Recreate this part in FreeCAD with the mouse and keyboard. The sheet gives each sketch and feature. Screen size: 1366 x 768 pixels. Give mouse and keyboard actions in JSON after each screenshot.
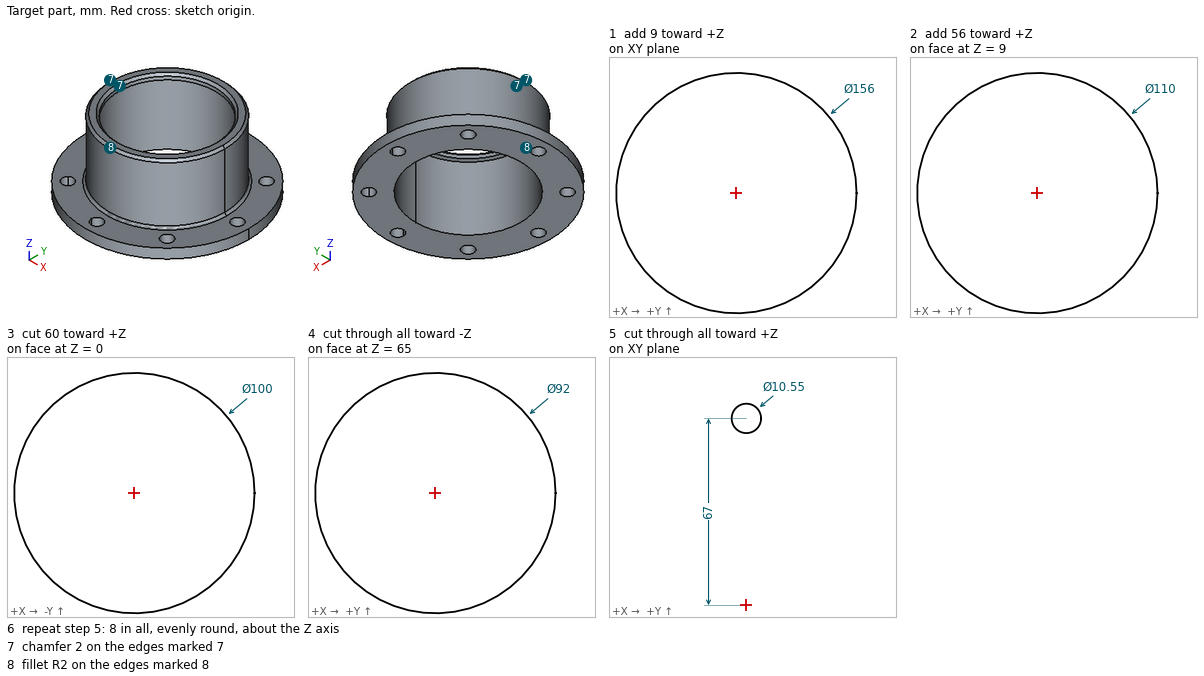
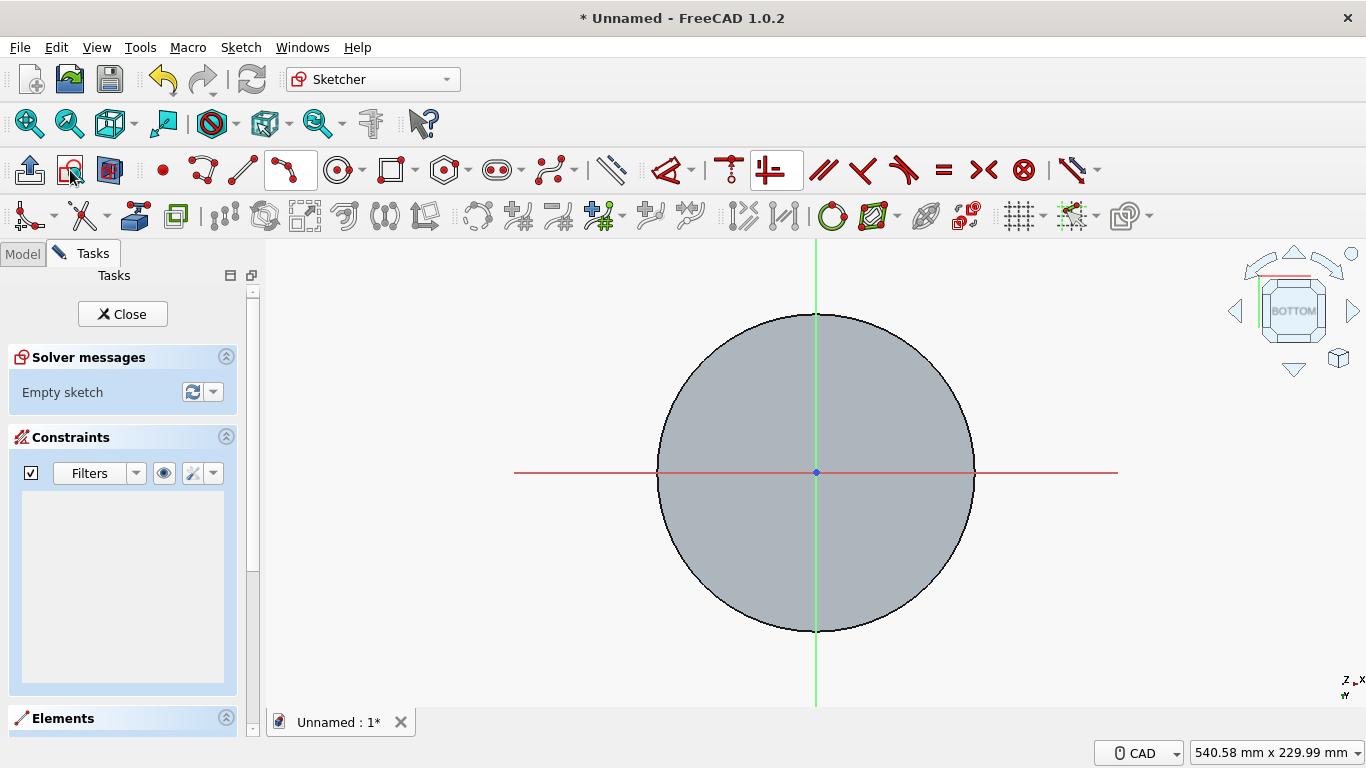
{"action": "scroll", "coordinate": [955, 473], "scroll_direction": "up", "scroll_amount": 2}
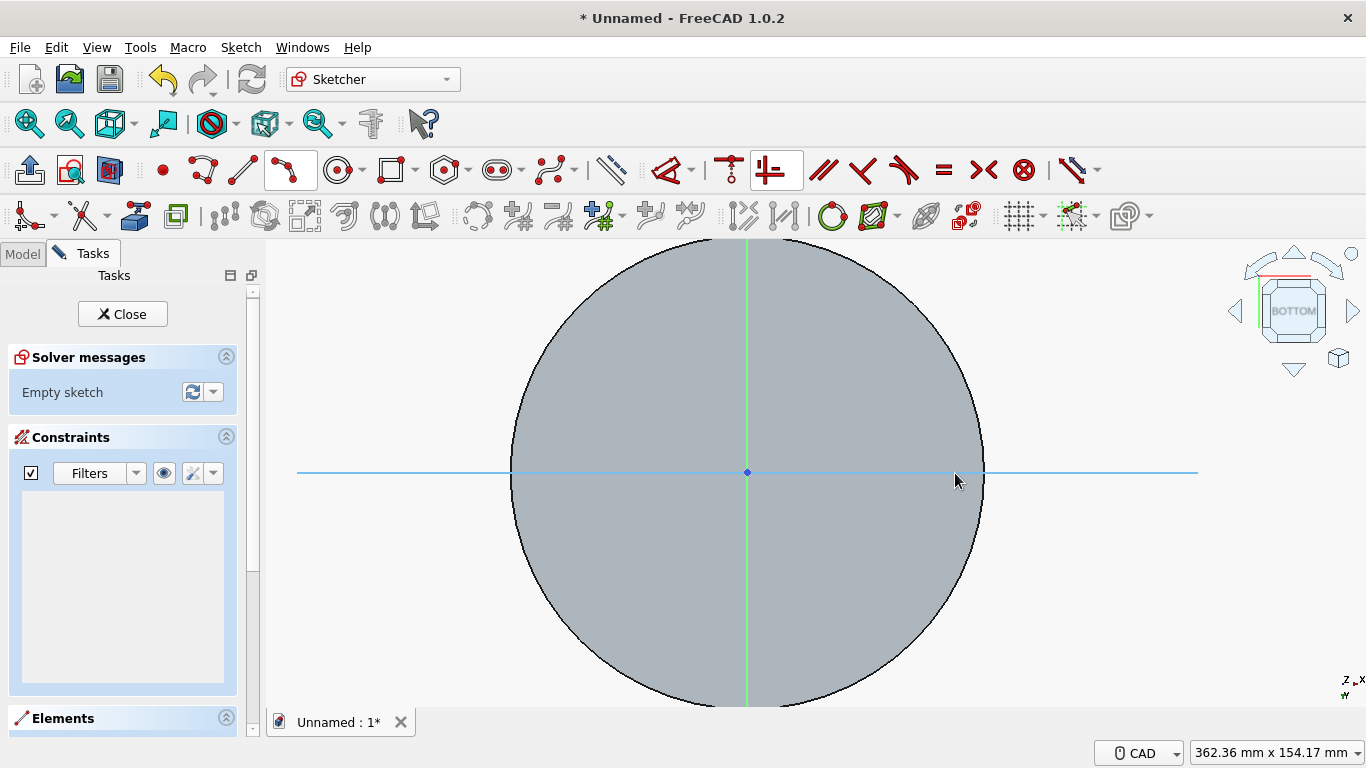
{"action": "left_click", "coordinate": [338, 170]}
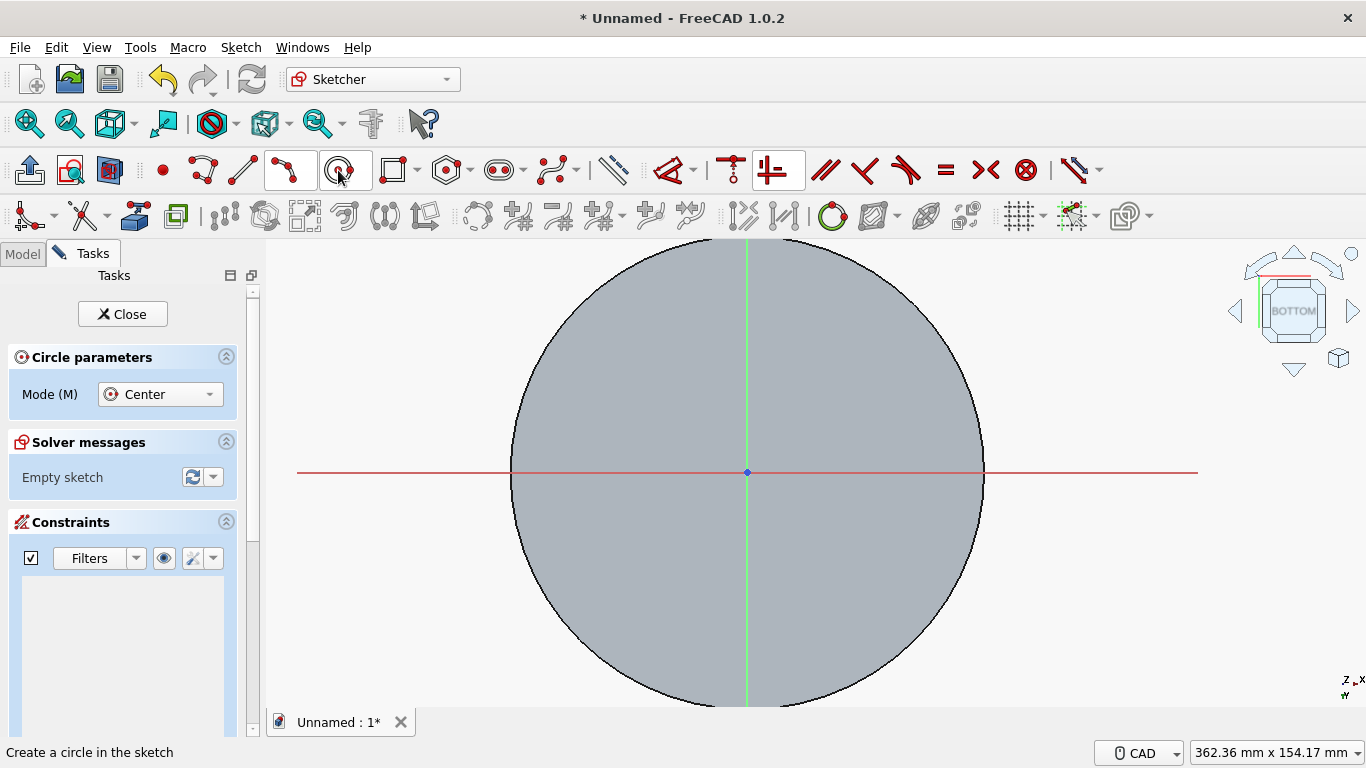
{"action": "left_click", "coordinate": [747, 473]}
{"action": "left_click", "coordinate": [855, 365]}
{"action": "key", "text": "Escape"}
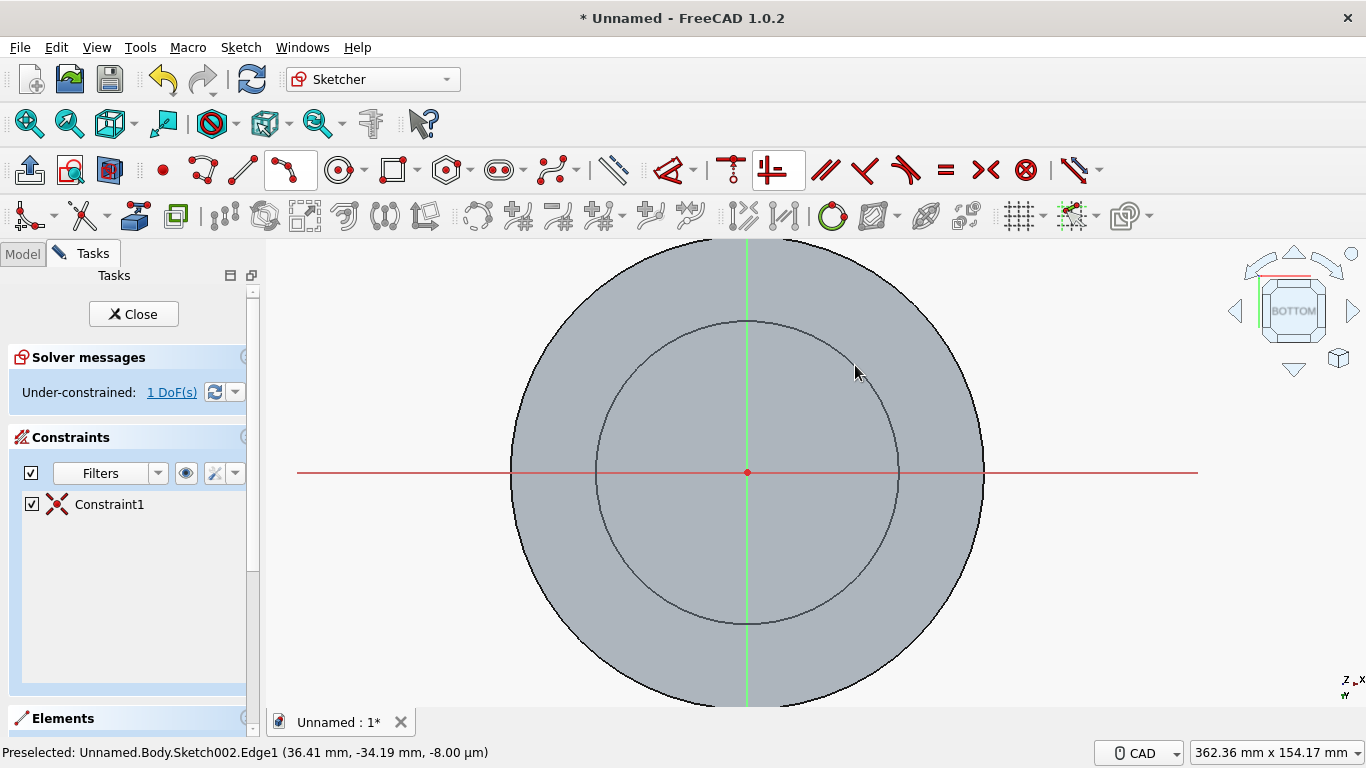
{"action": "left_click", "coordinate": [668, 170]}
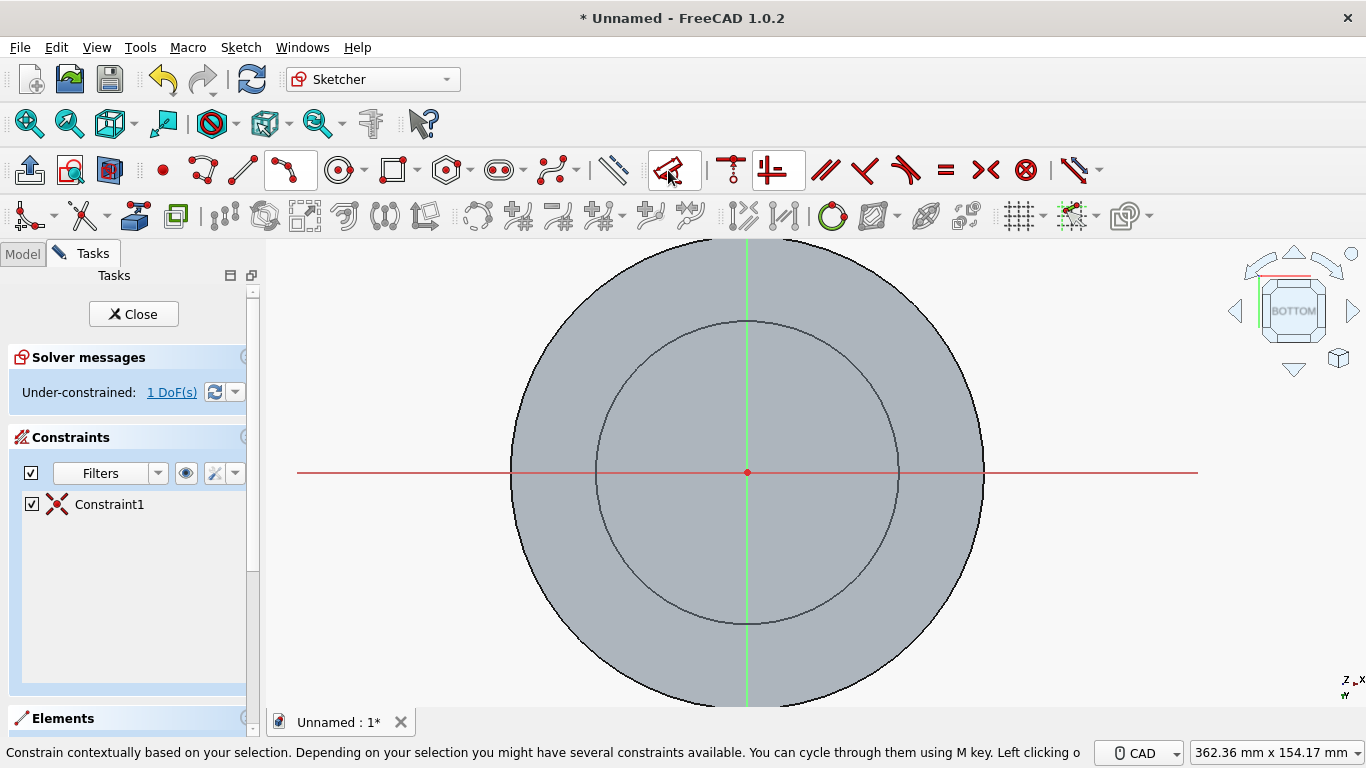
{"action": "left_click", "coordinate": [854, 365]}
{"action": "left_click", "coordinate": [877, 342]}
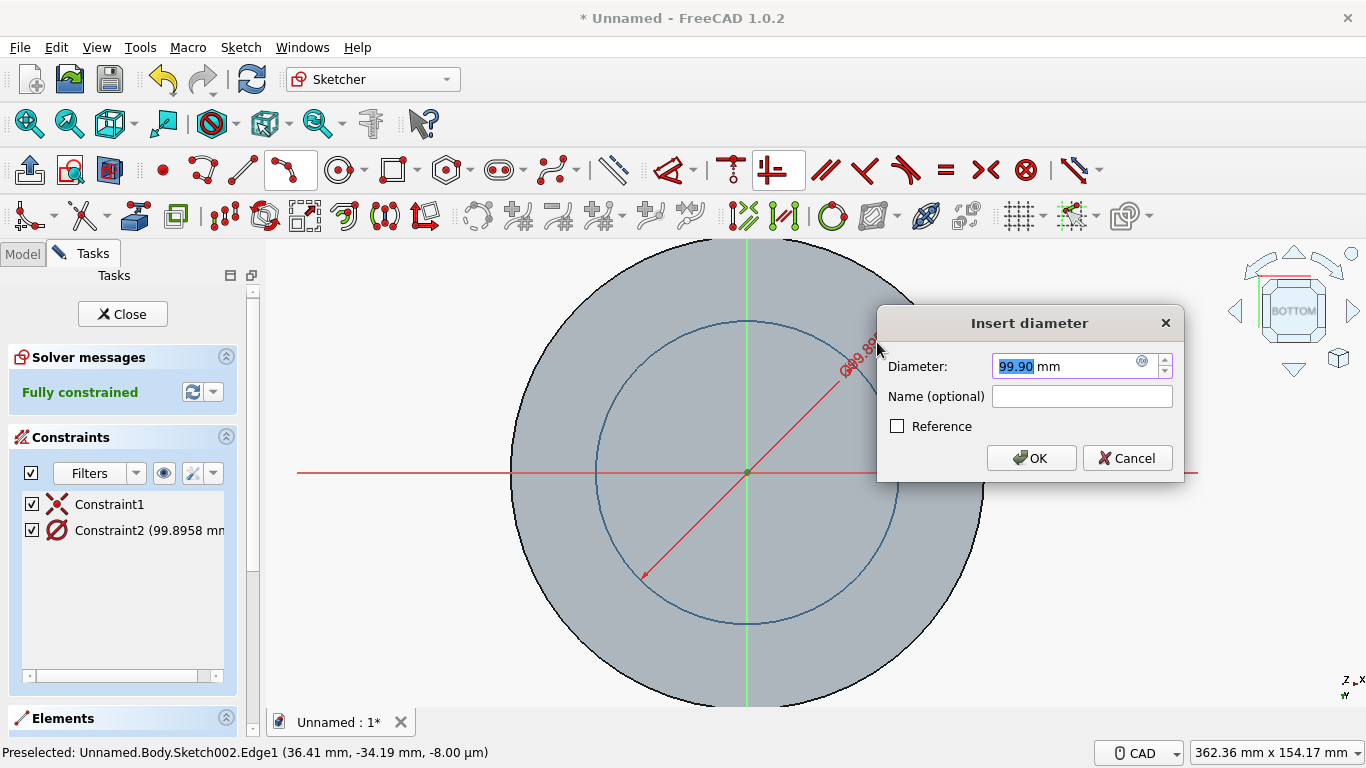
{"action": "type", "text": "100"}
{"action": "key", "text": "Return"}
{"action": "key", "text": "Escape"}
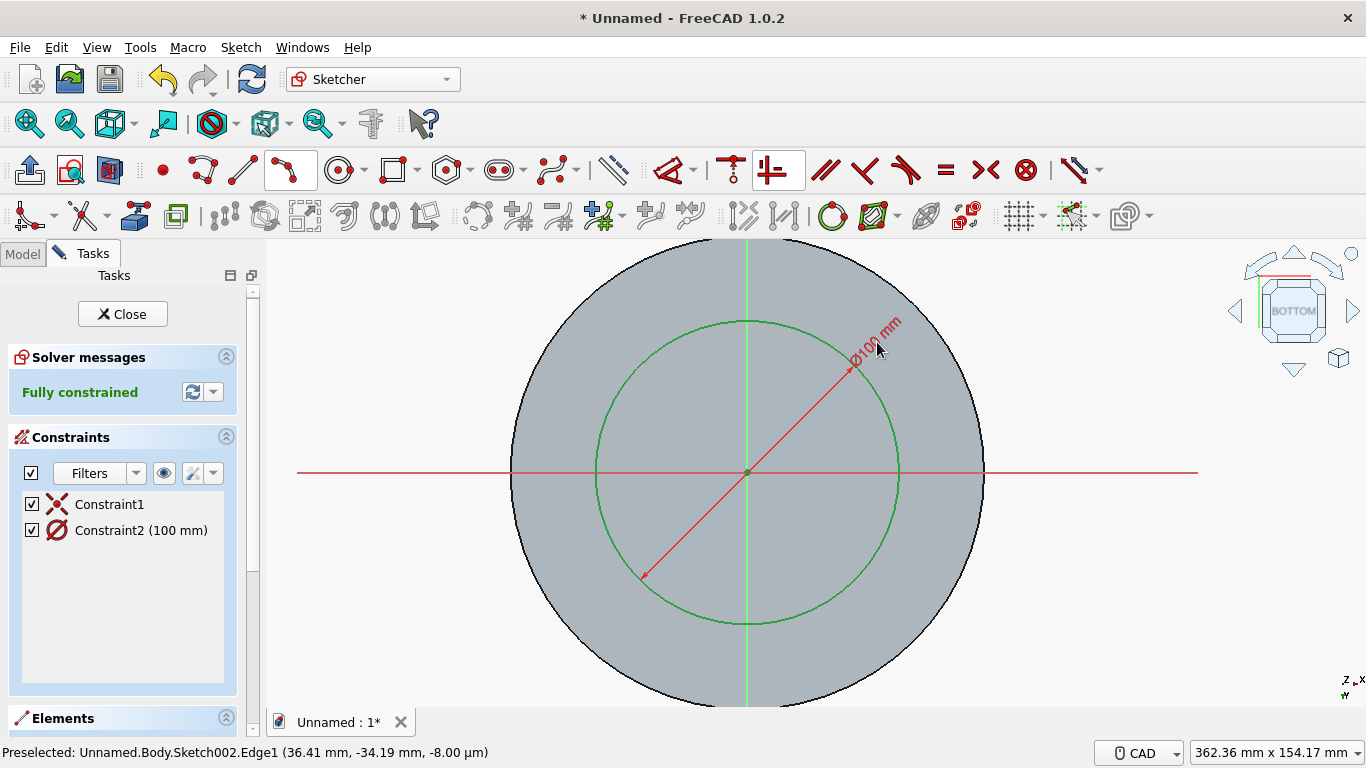
{"action": "left_click", "coordinate": [123, 314]}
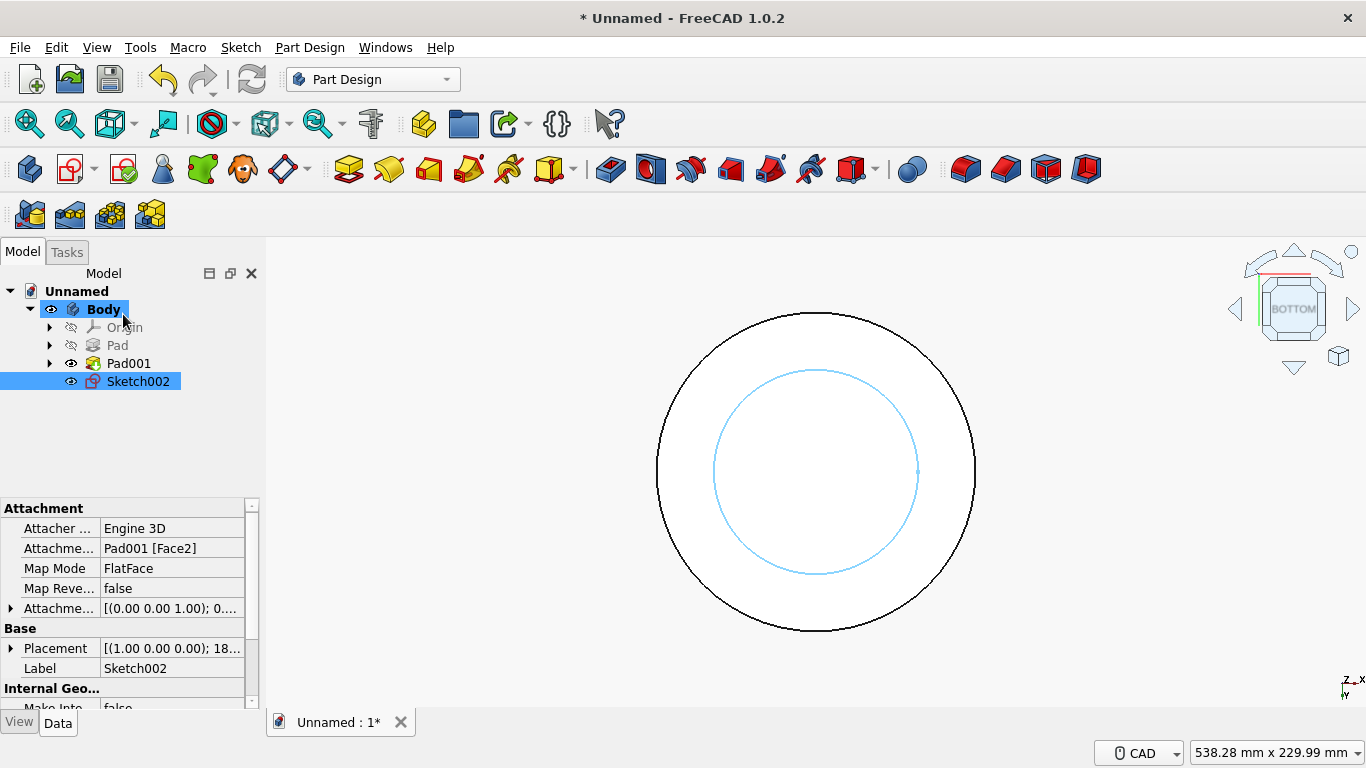
{"action": "left_click", "coordinate": [612, 170]}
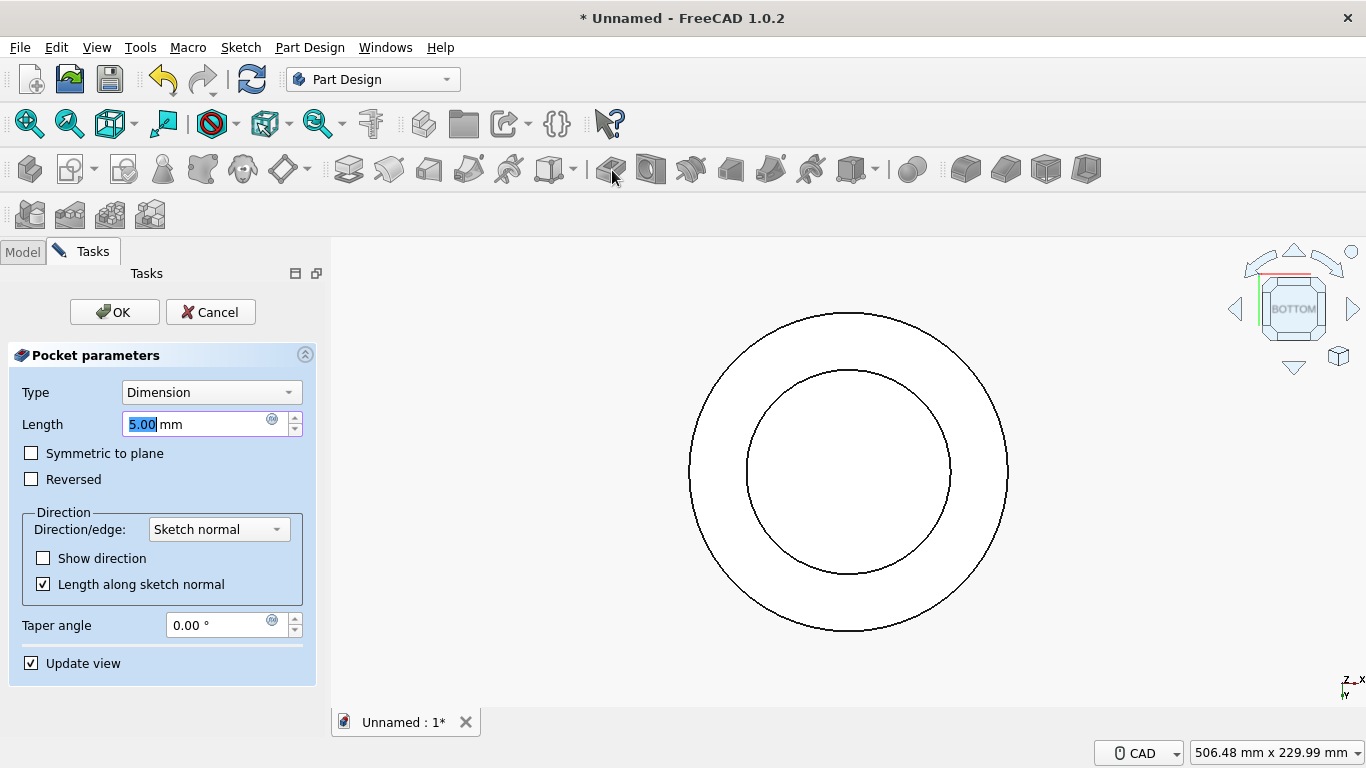
{"action": "type", "text": "60"}
{"action": "key", "text": "Tab"}